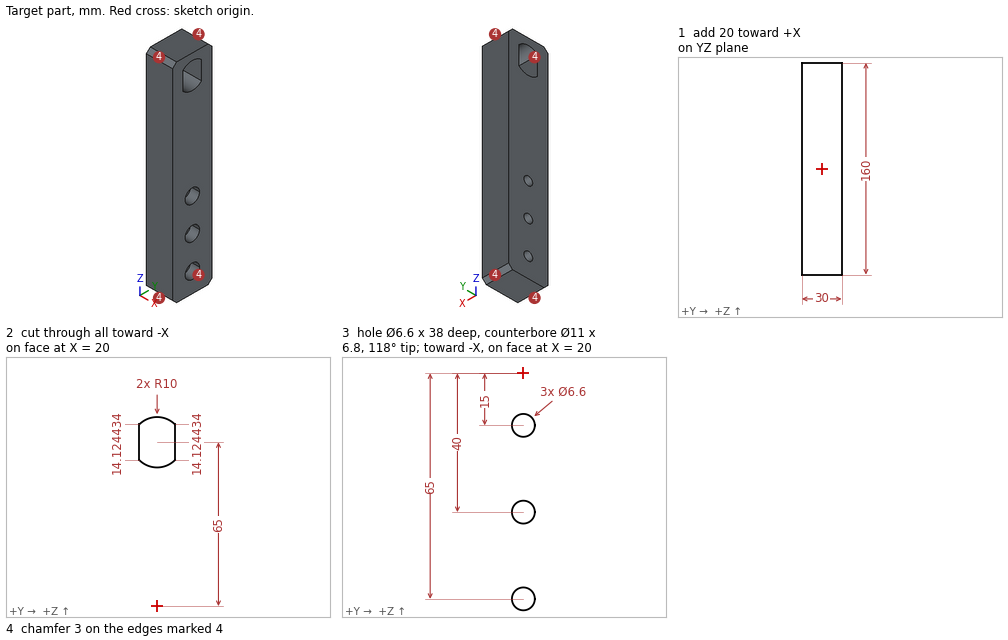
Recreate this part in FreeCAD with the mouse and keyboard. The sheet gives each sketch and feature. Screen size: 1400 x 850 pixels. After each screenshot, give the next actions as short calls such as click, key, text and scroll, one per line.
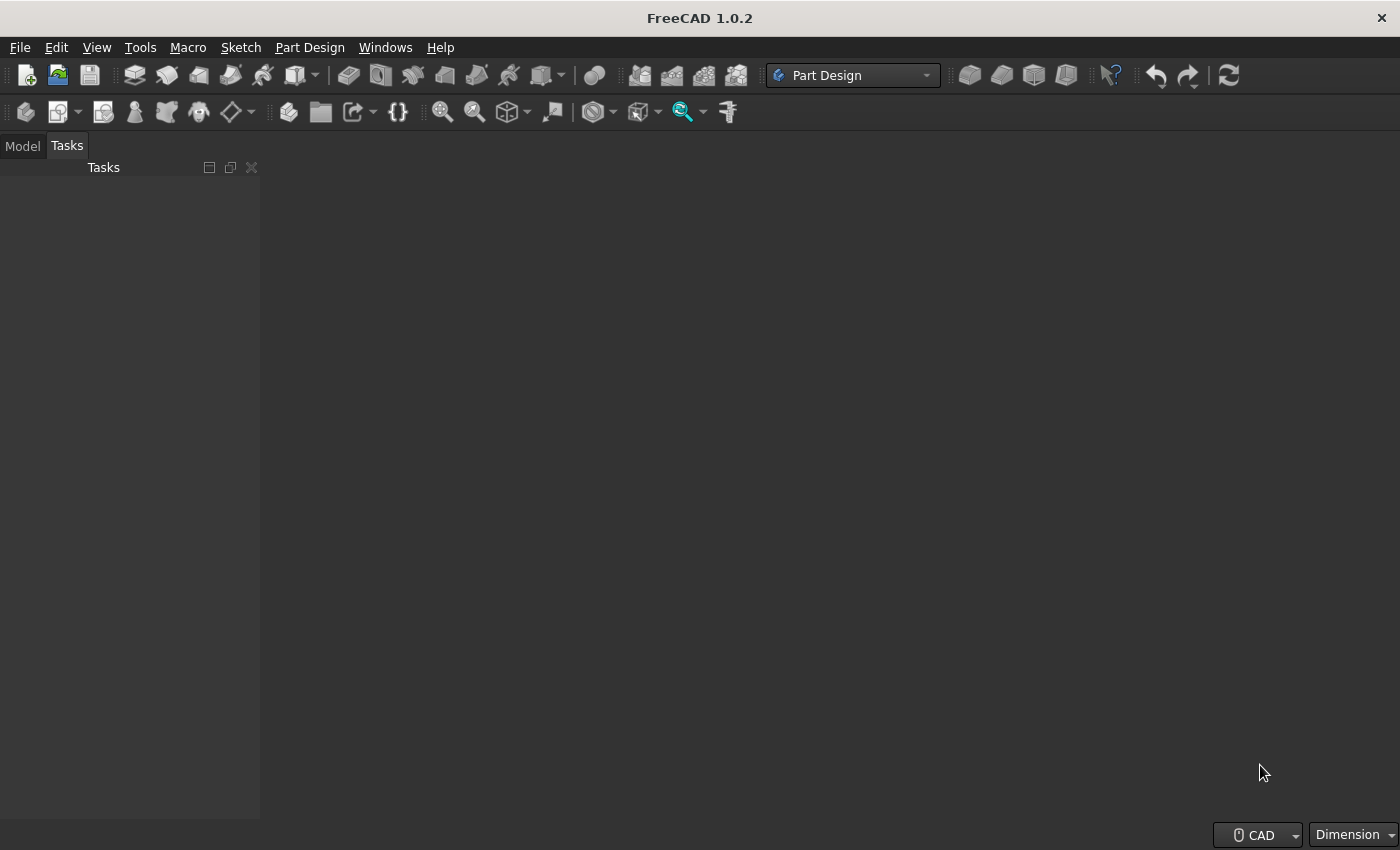
key(ctrl+n)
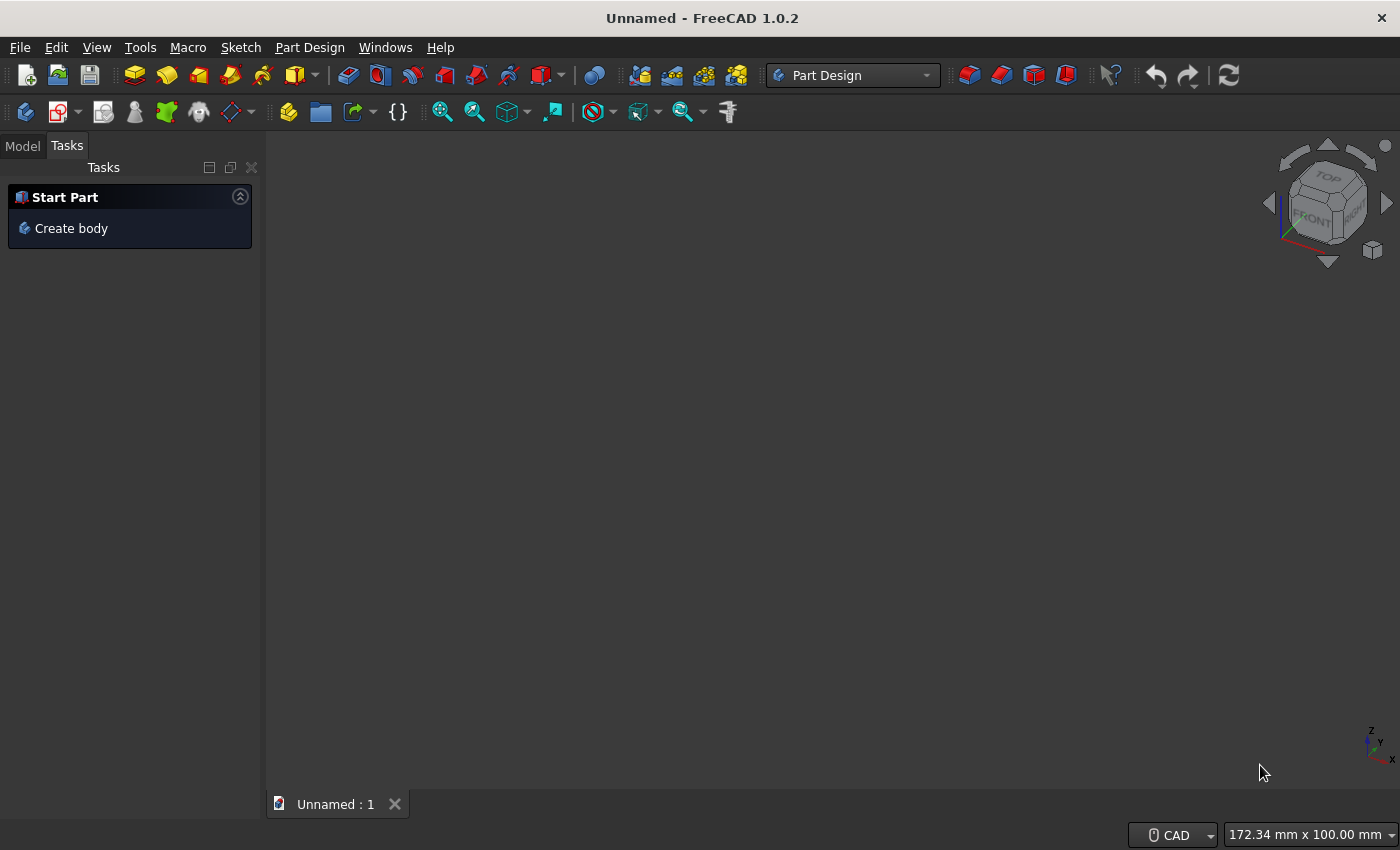
click(58, 112)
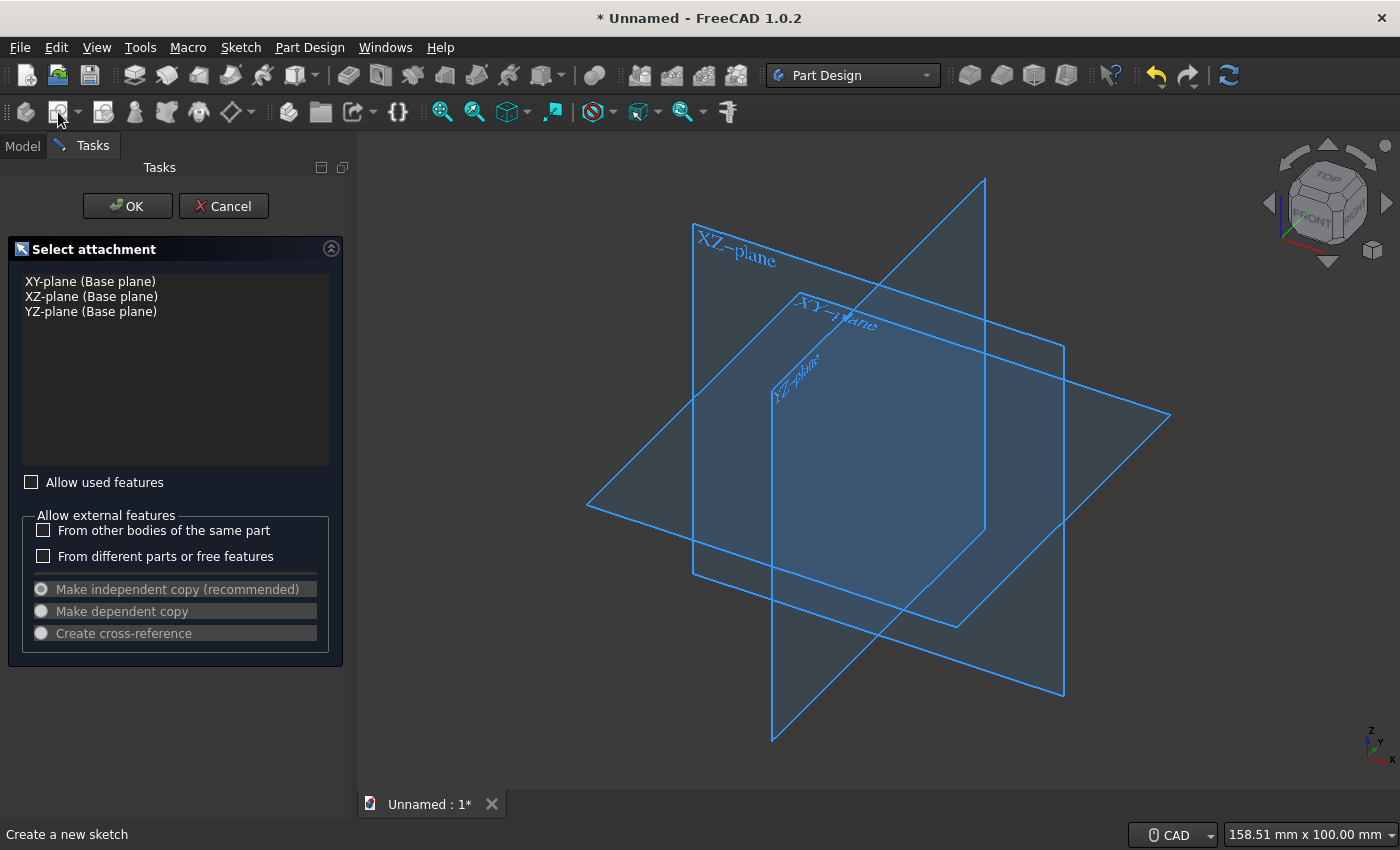
click(82, 312)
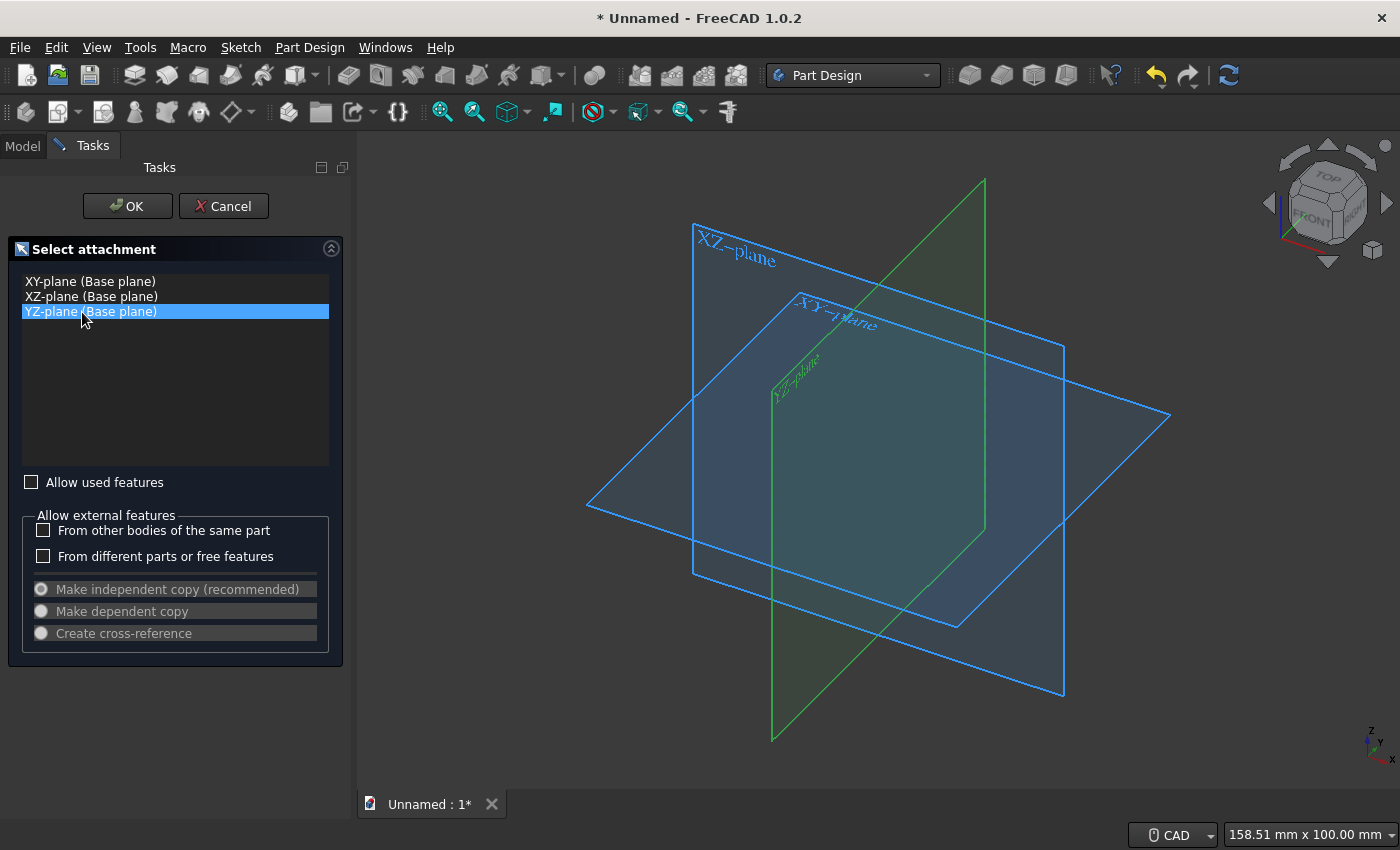
click(128, 206)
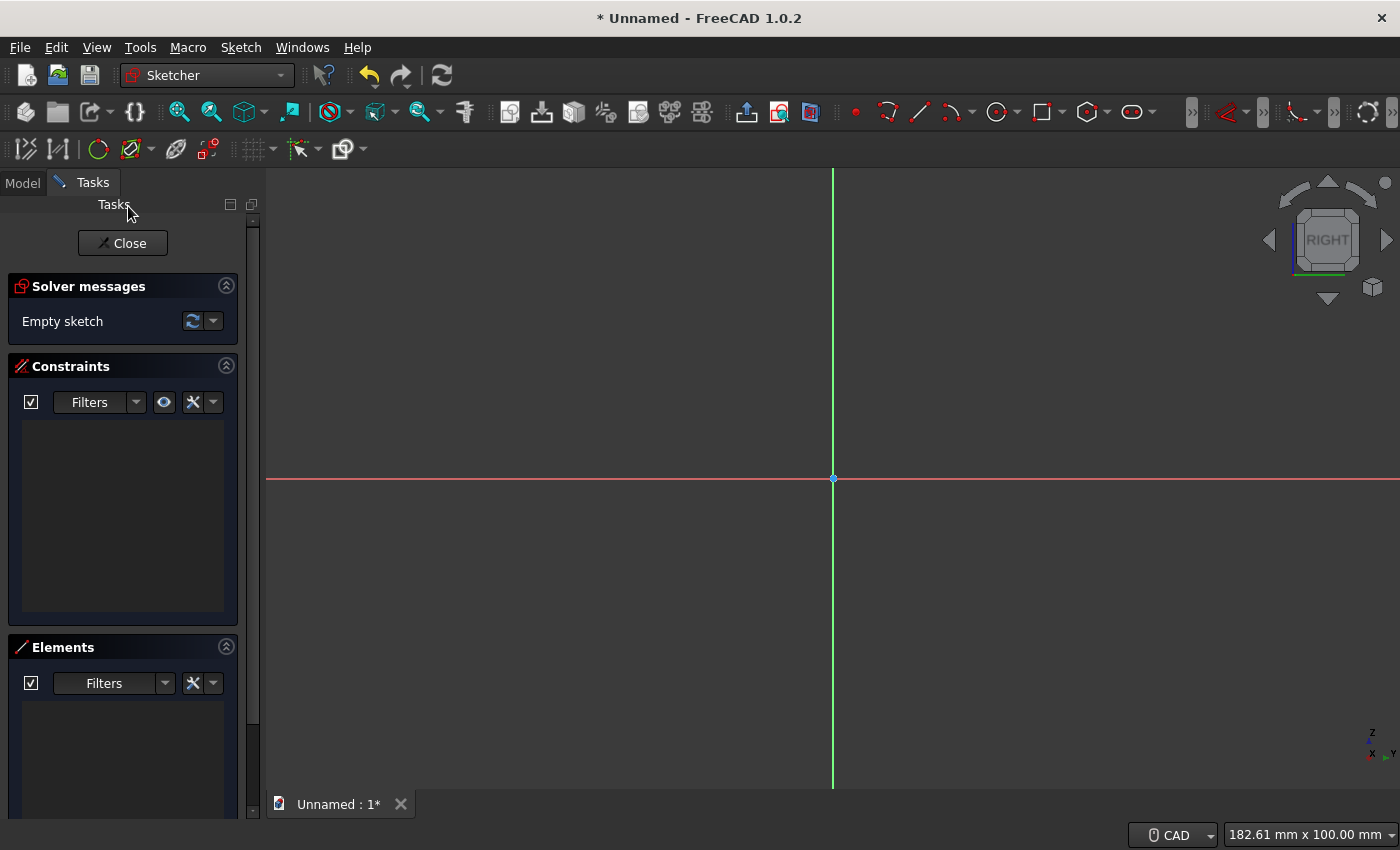
scroll(725, 479, down, 5)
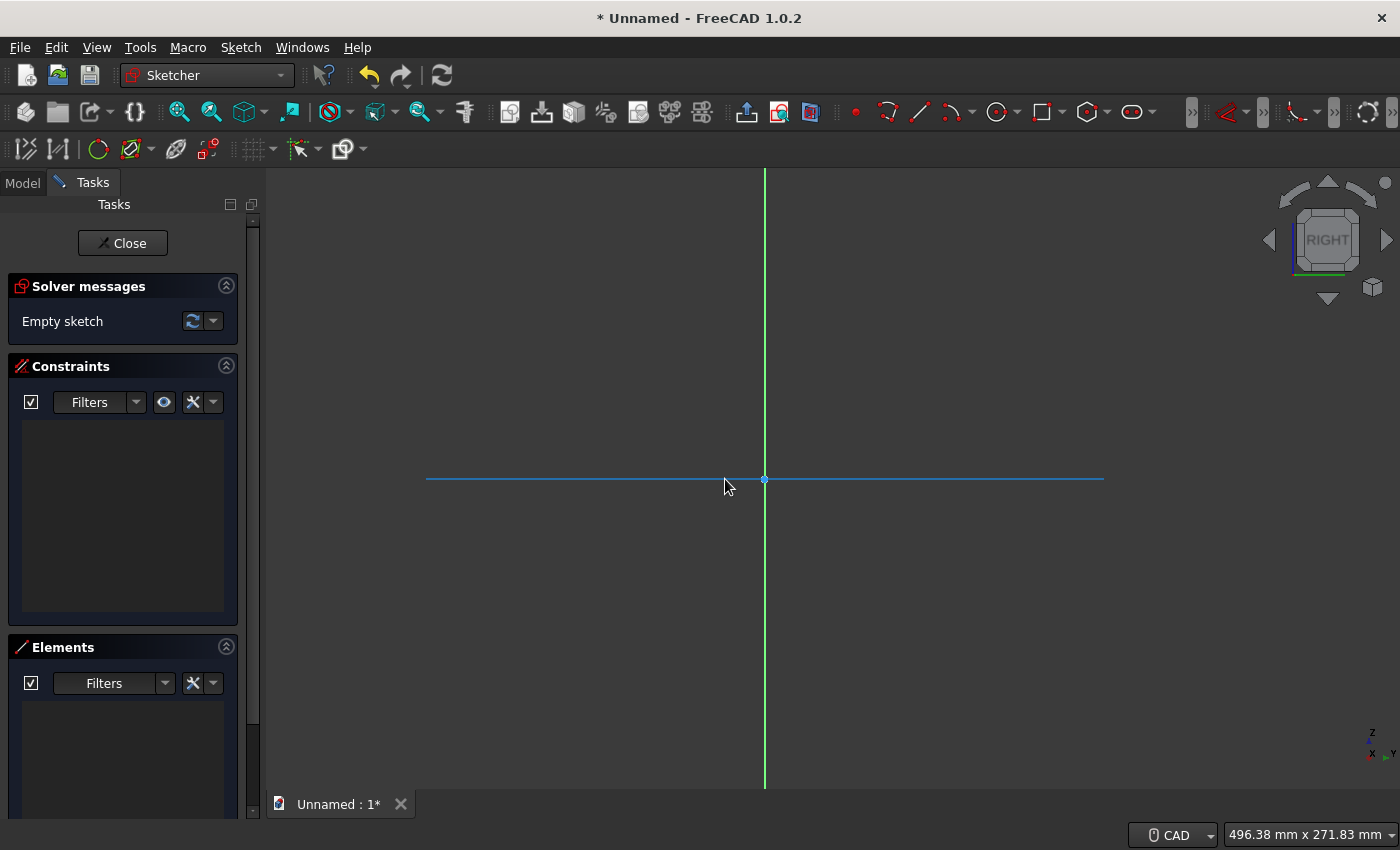
key(g)
key(v)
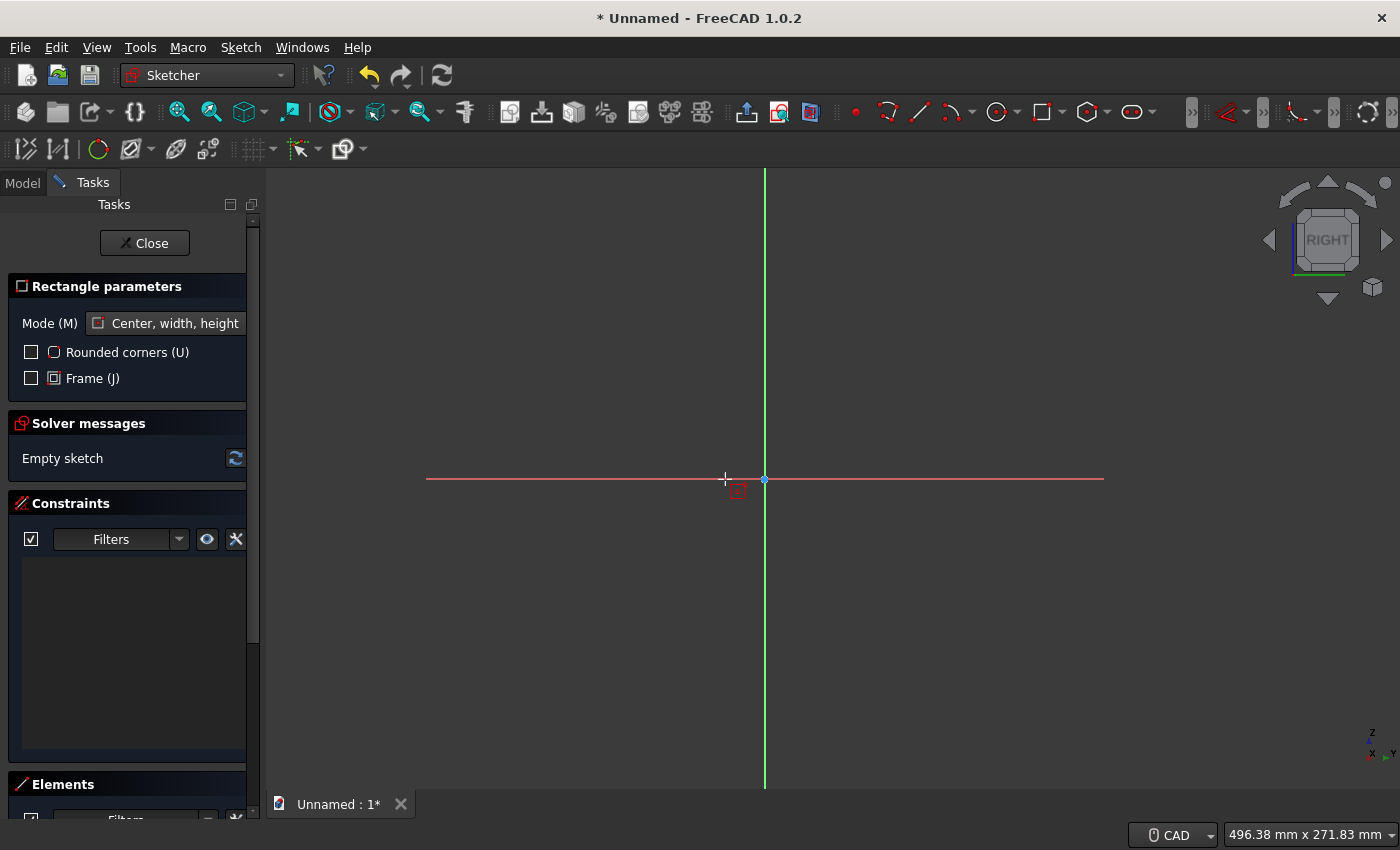
click(765, 479)
move(799, 296)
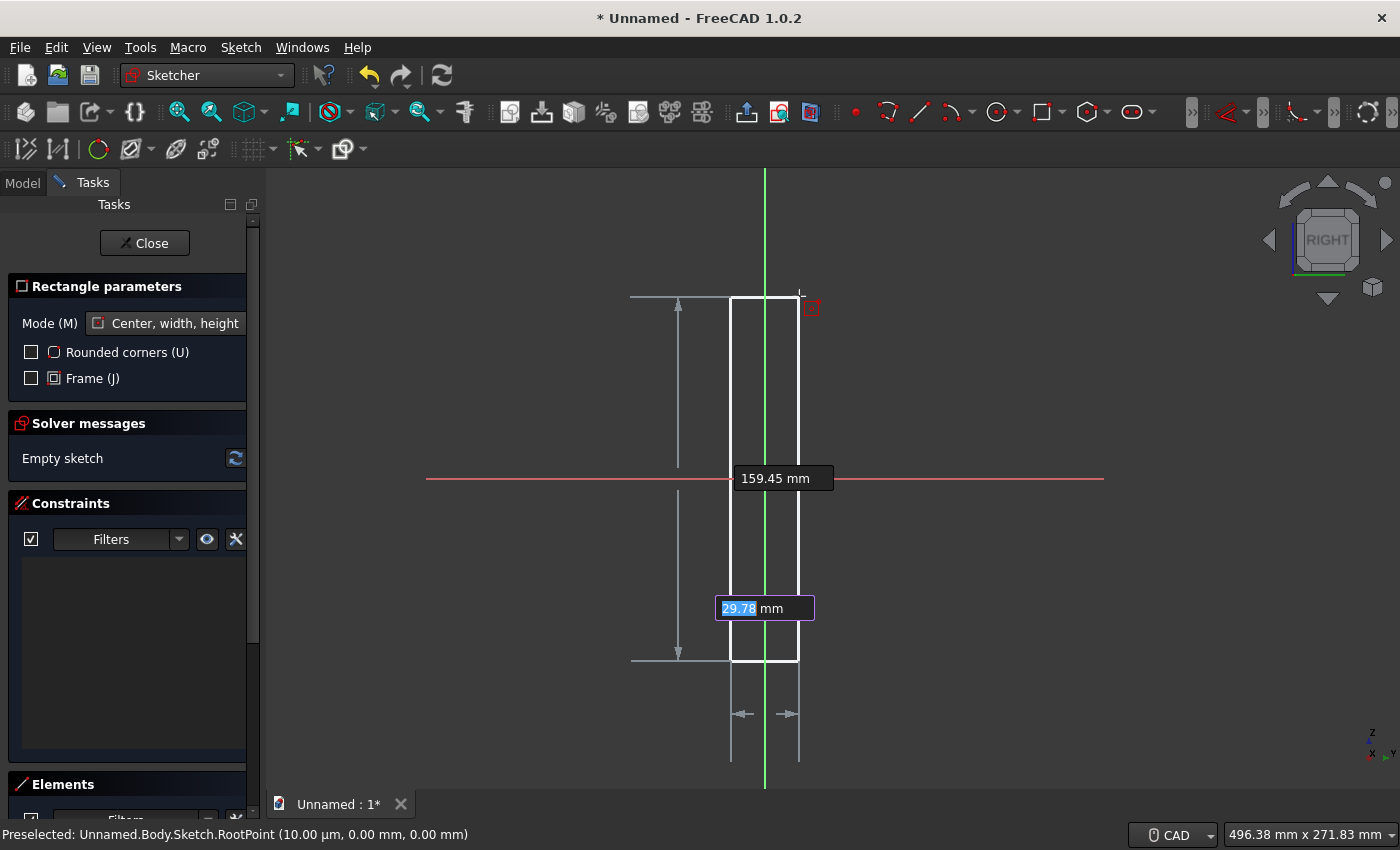
text(30)
key(Tab)
text(160)
key(Return)
key(Escape)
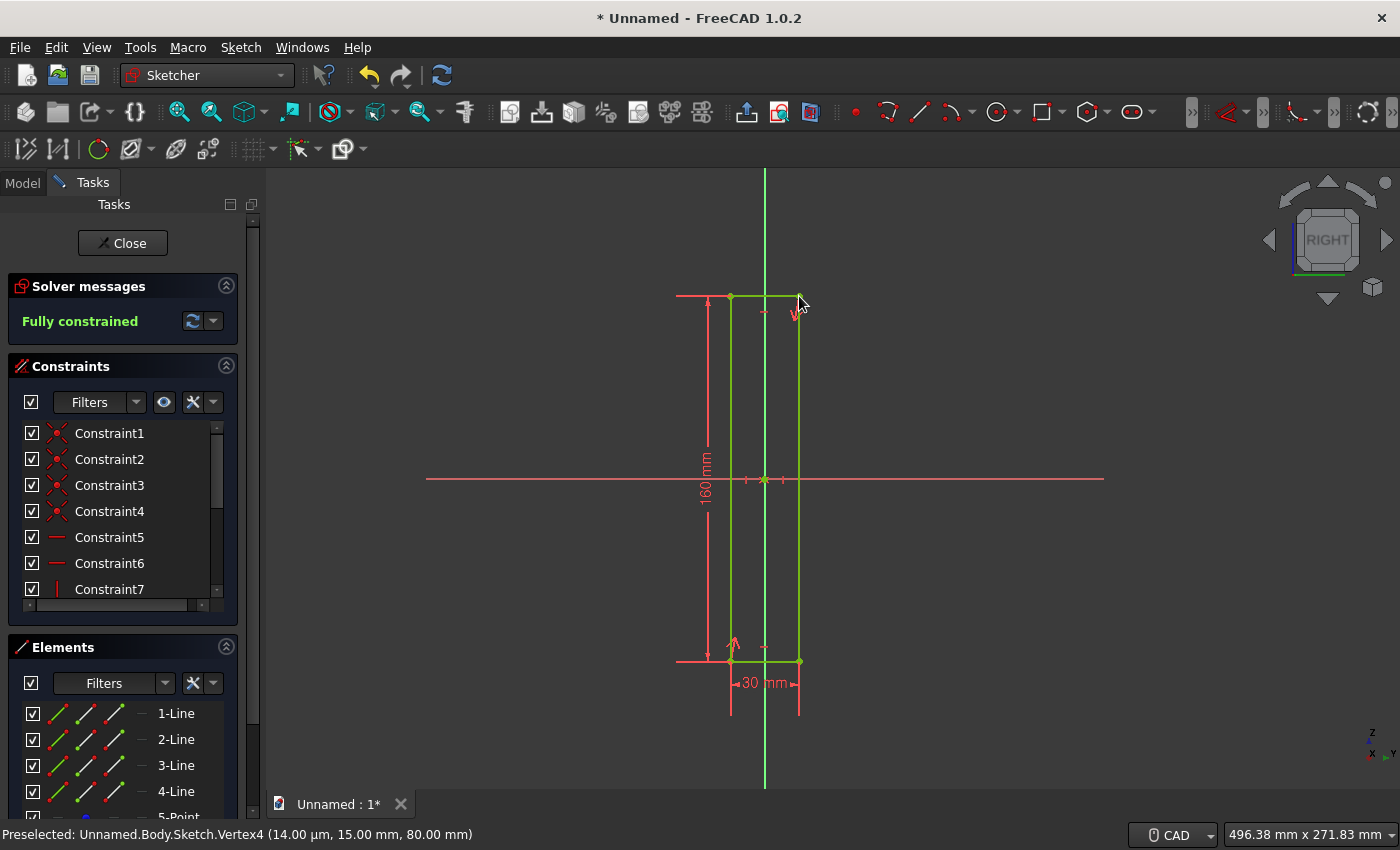
click(123, 243)